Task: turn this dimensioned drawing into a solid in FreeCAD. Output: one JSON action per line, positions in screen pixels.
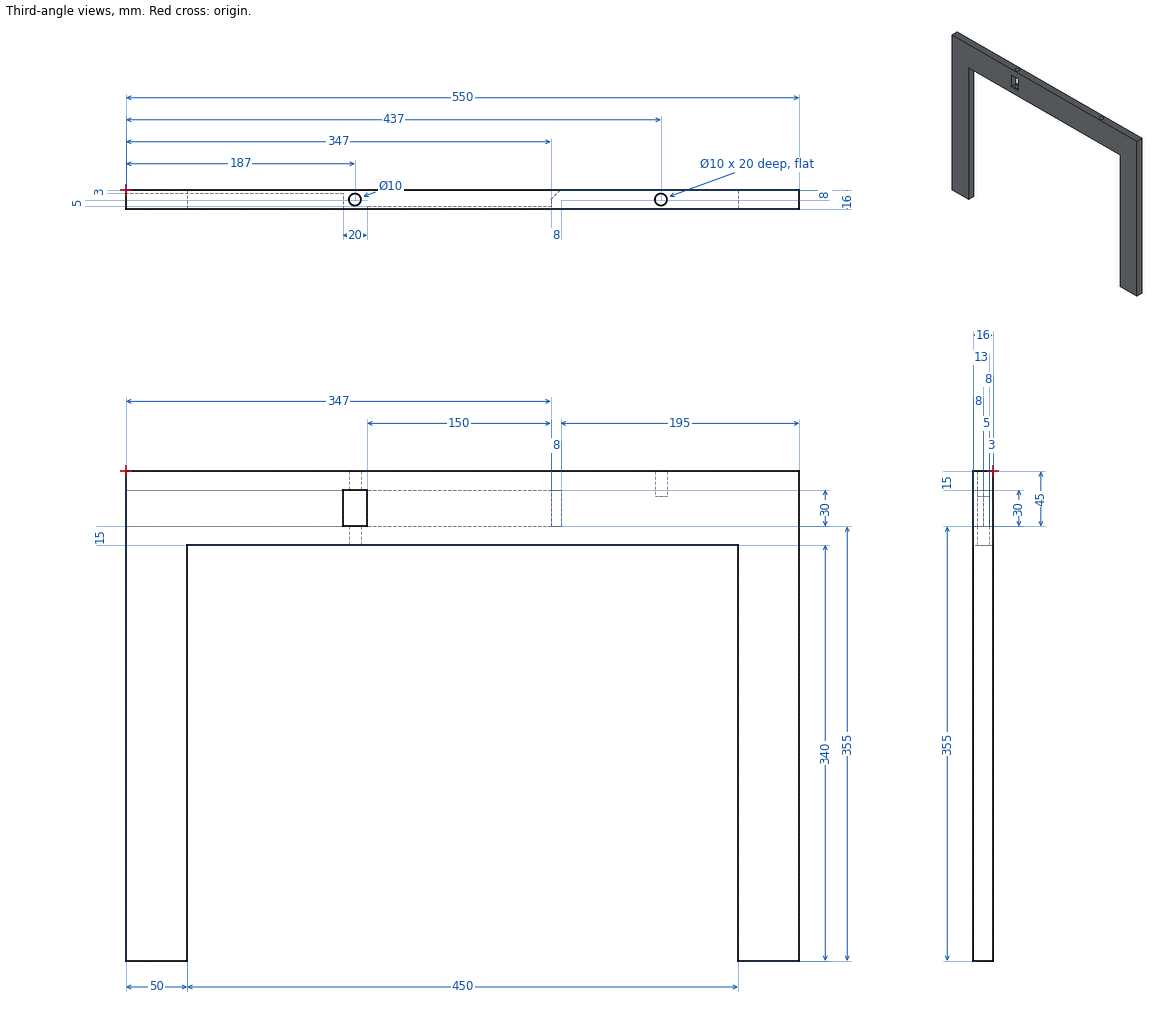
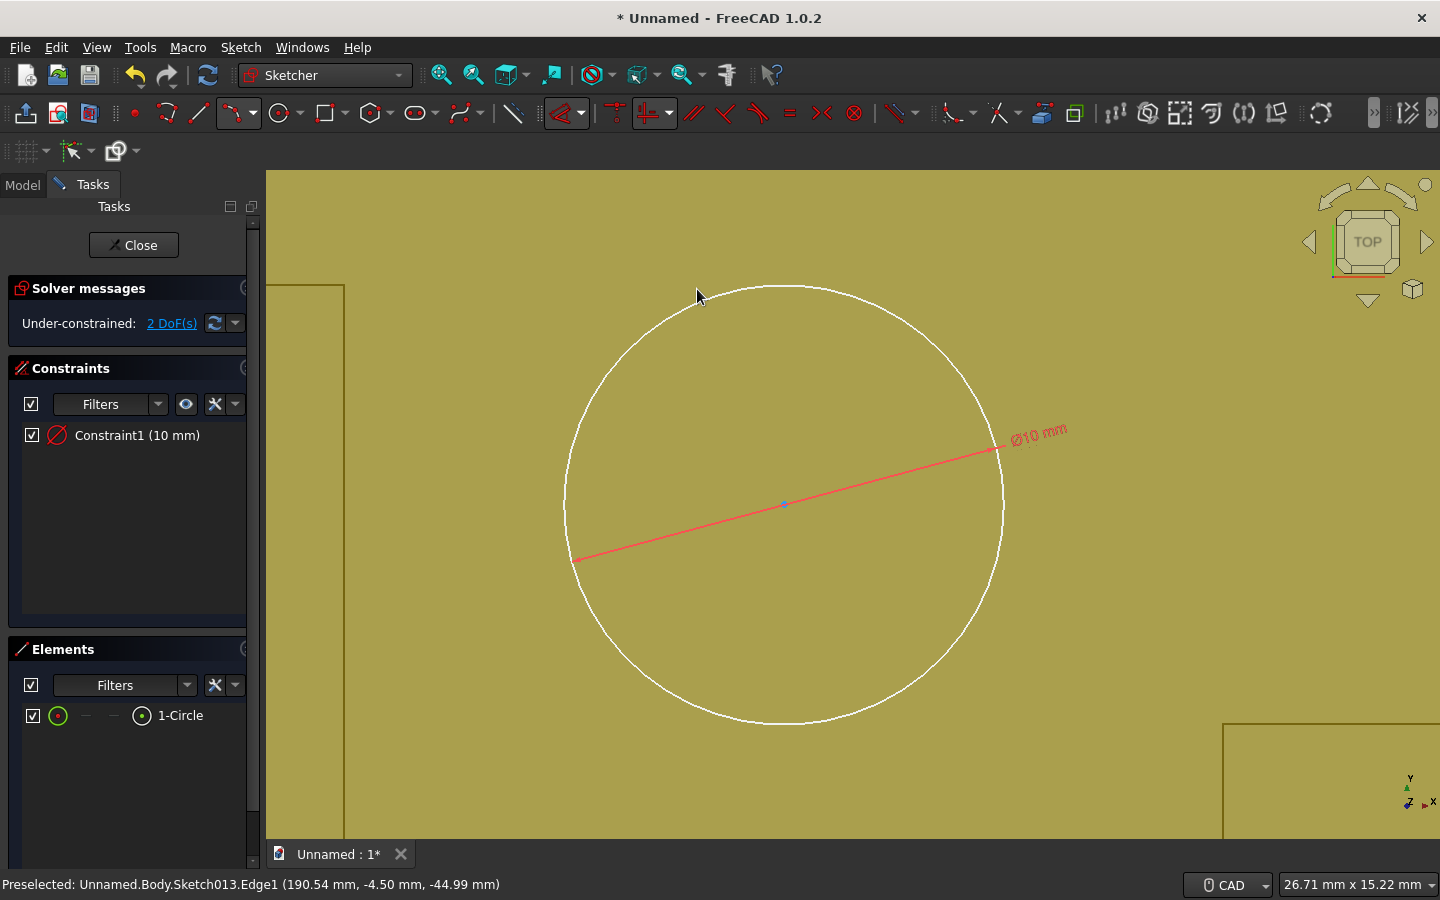
{"action": "left_click", "coordinate": [784, 505]}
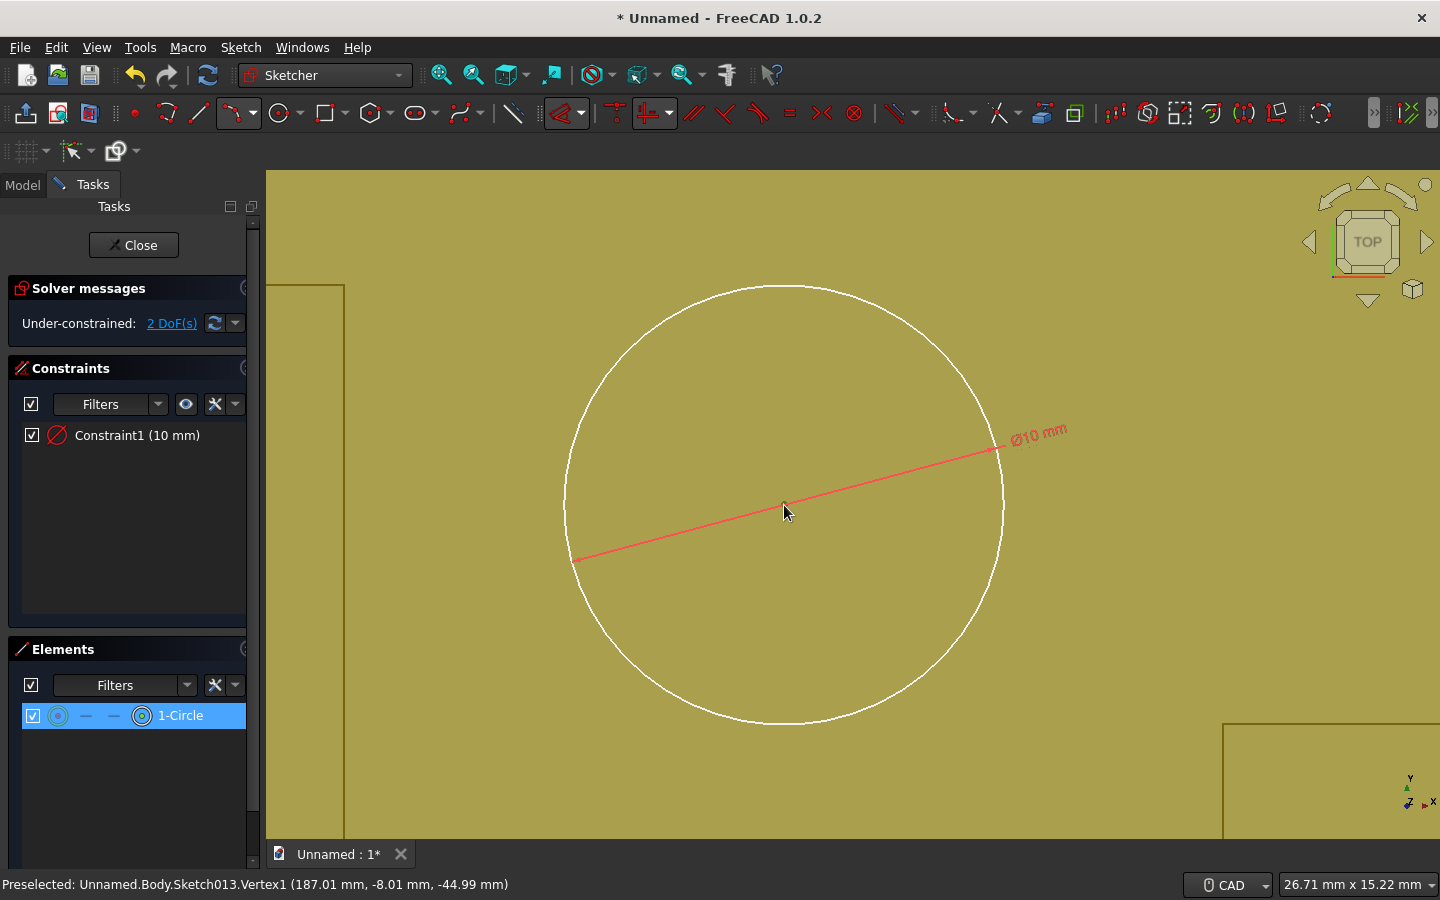
{"action": "key", "text": "i"}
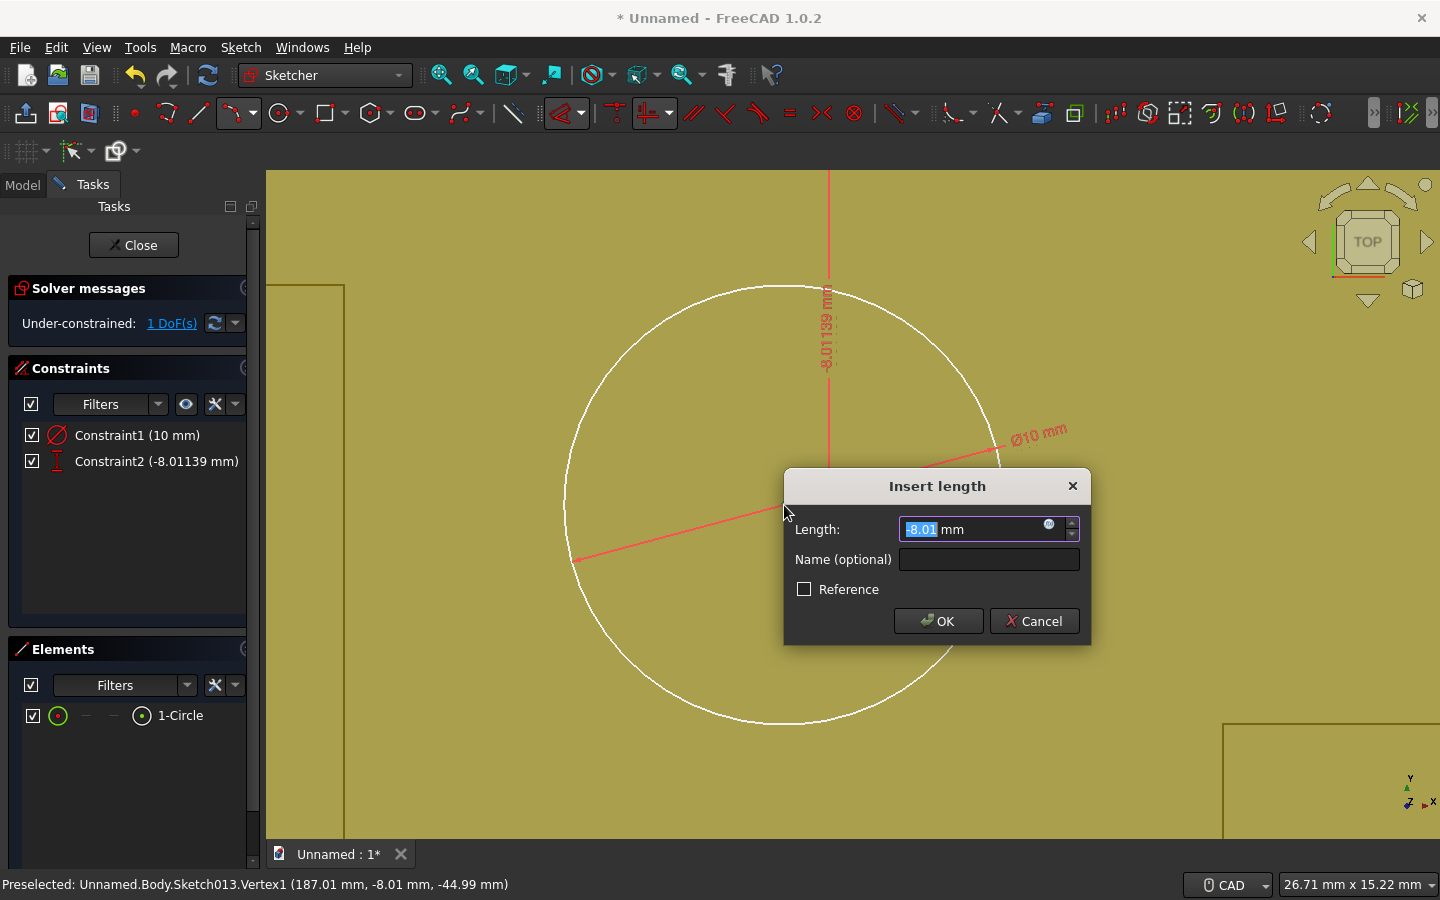
{"action": "type", "text": "-8"}
{"action": "key", "text": "Return"}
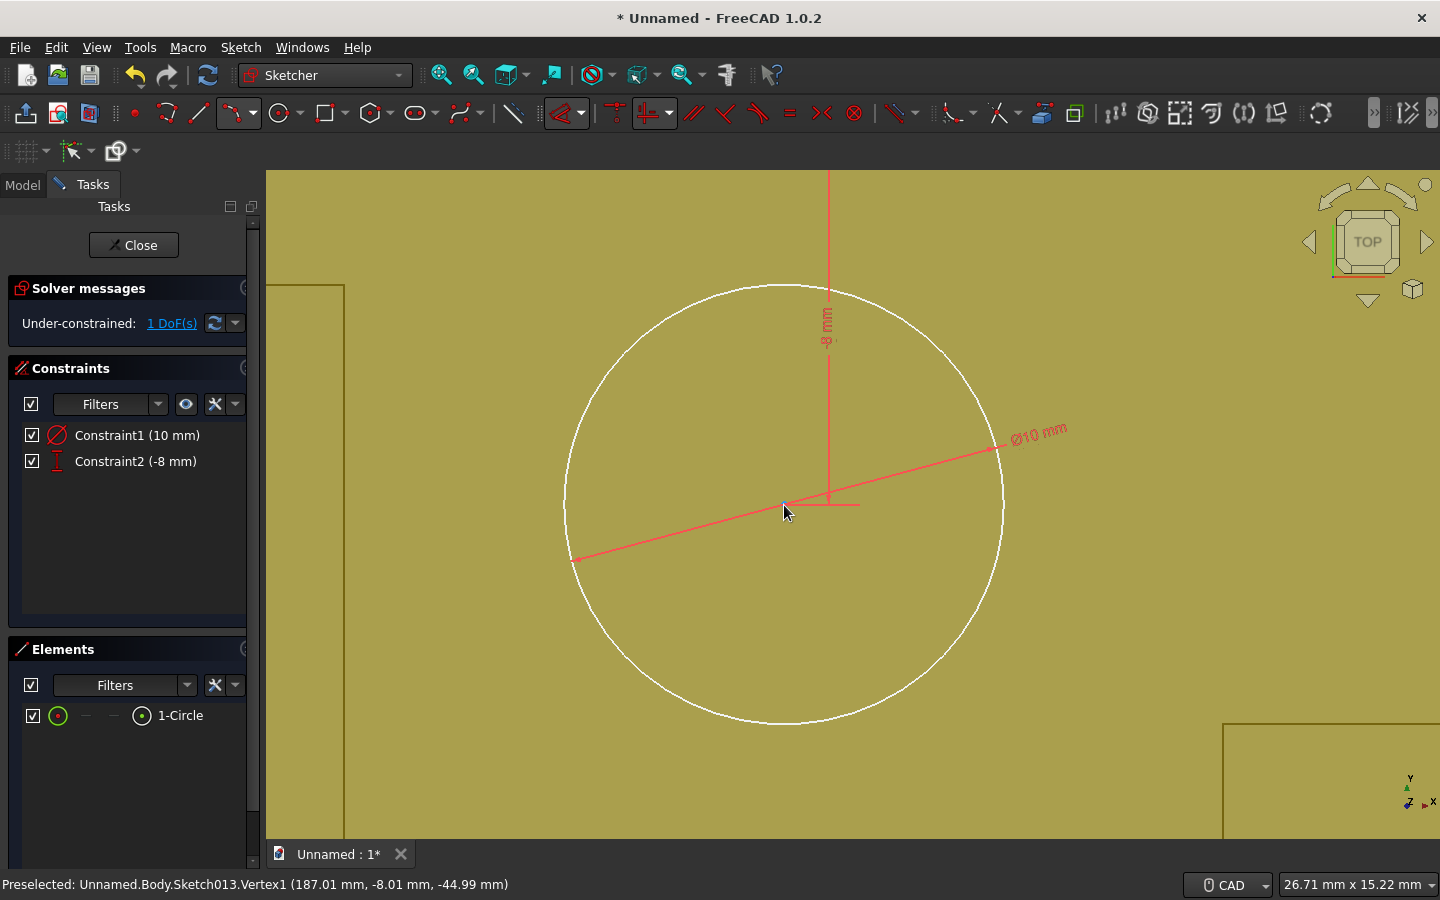
{"action": "left_click", "coordinate": [784, 504]}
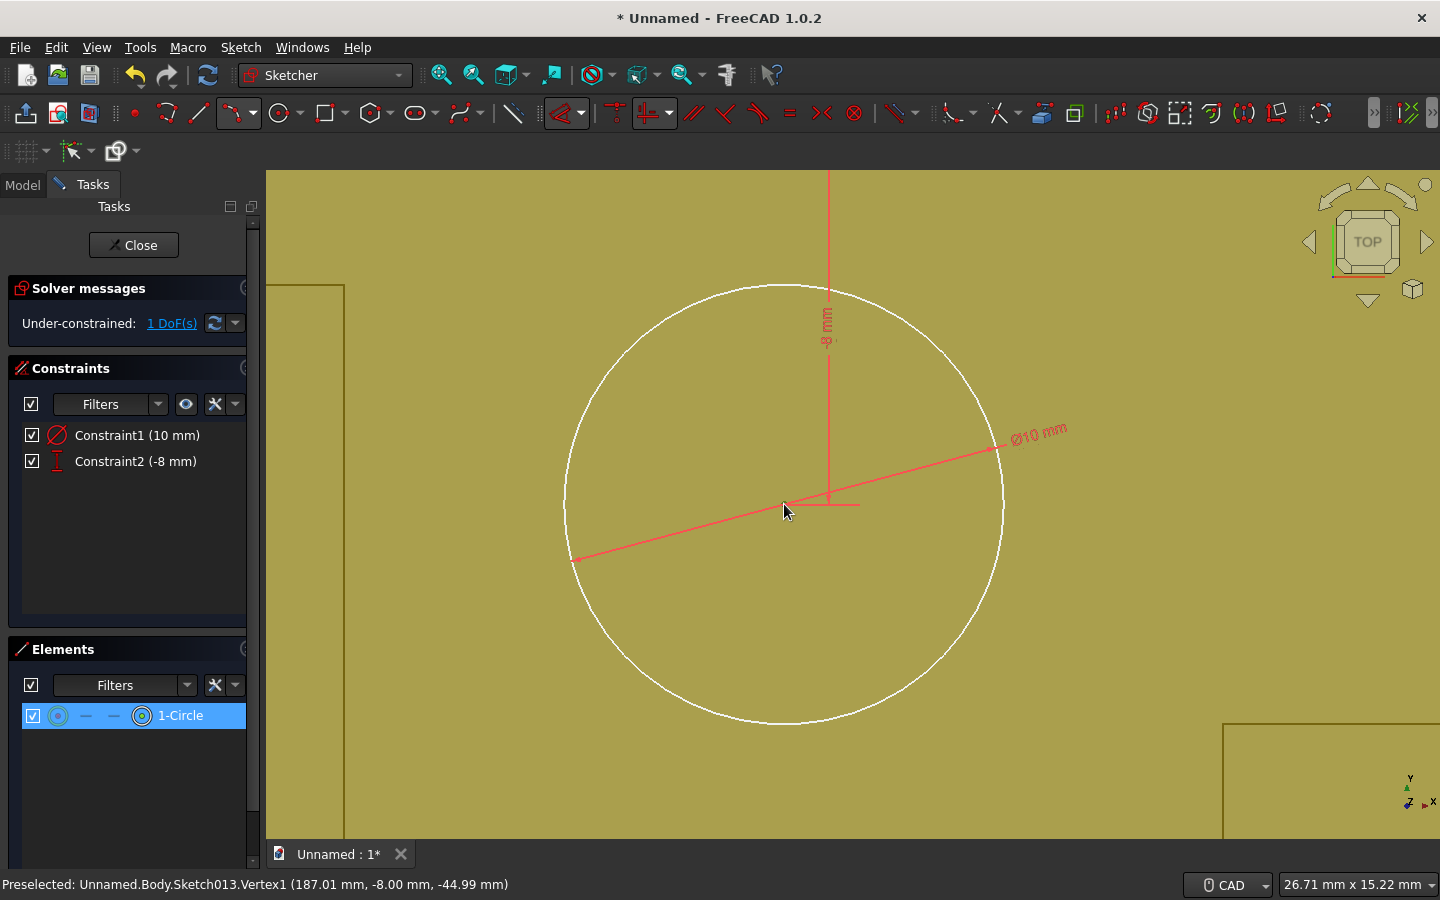
{"action": "key", "text": "l"}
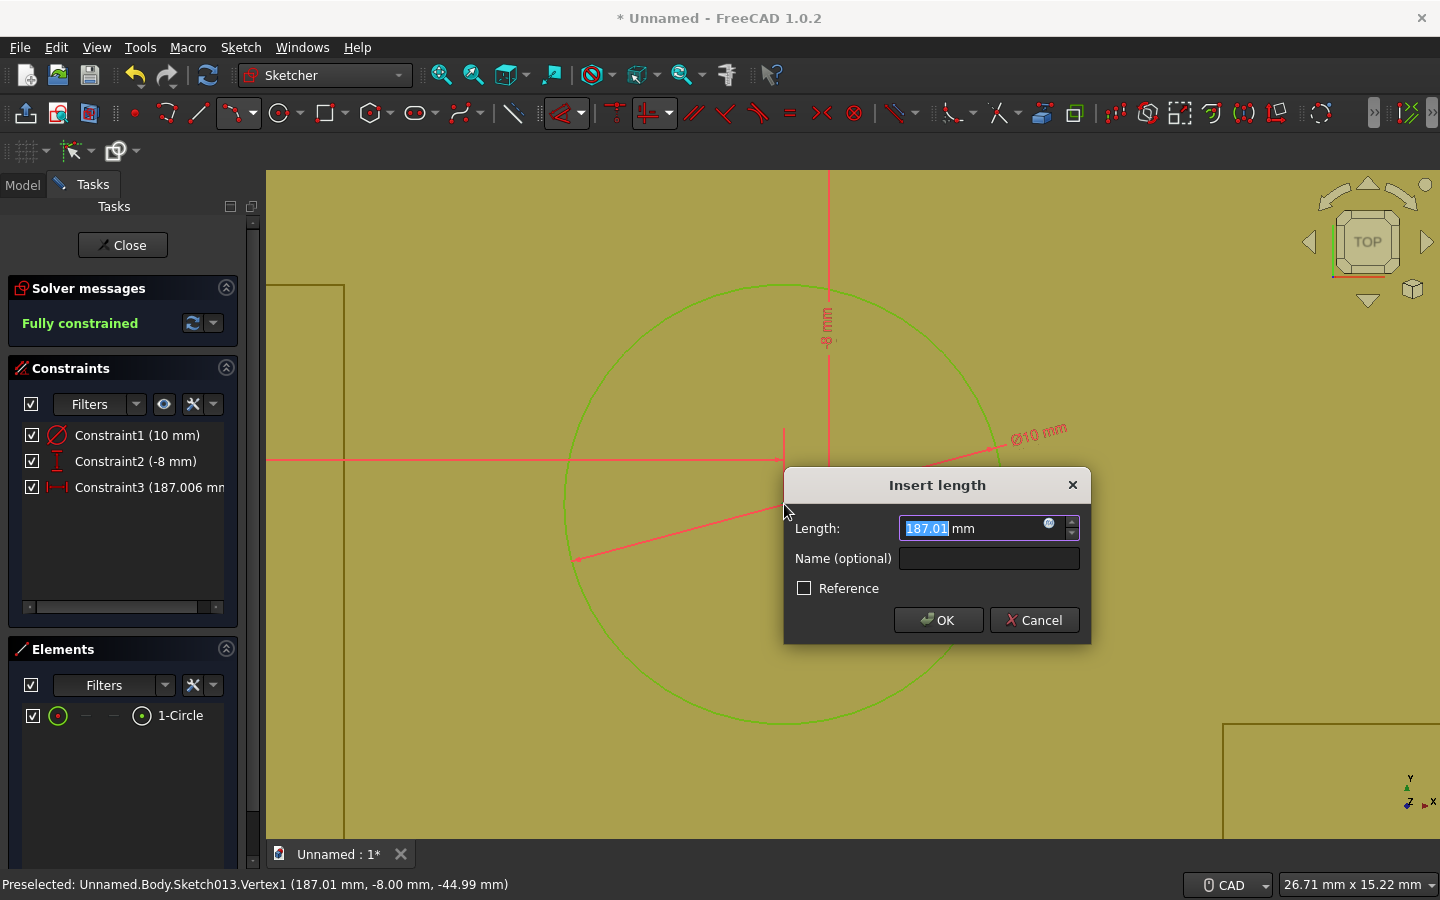
{"action": "type", "text": "187"}
{"action": "key", "text": "Return"}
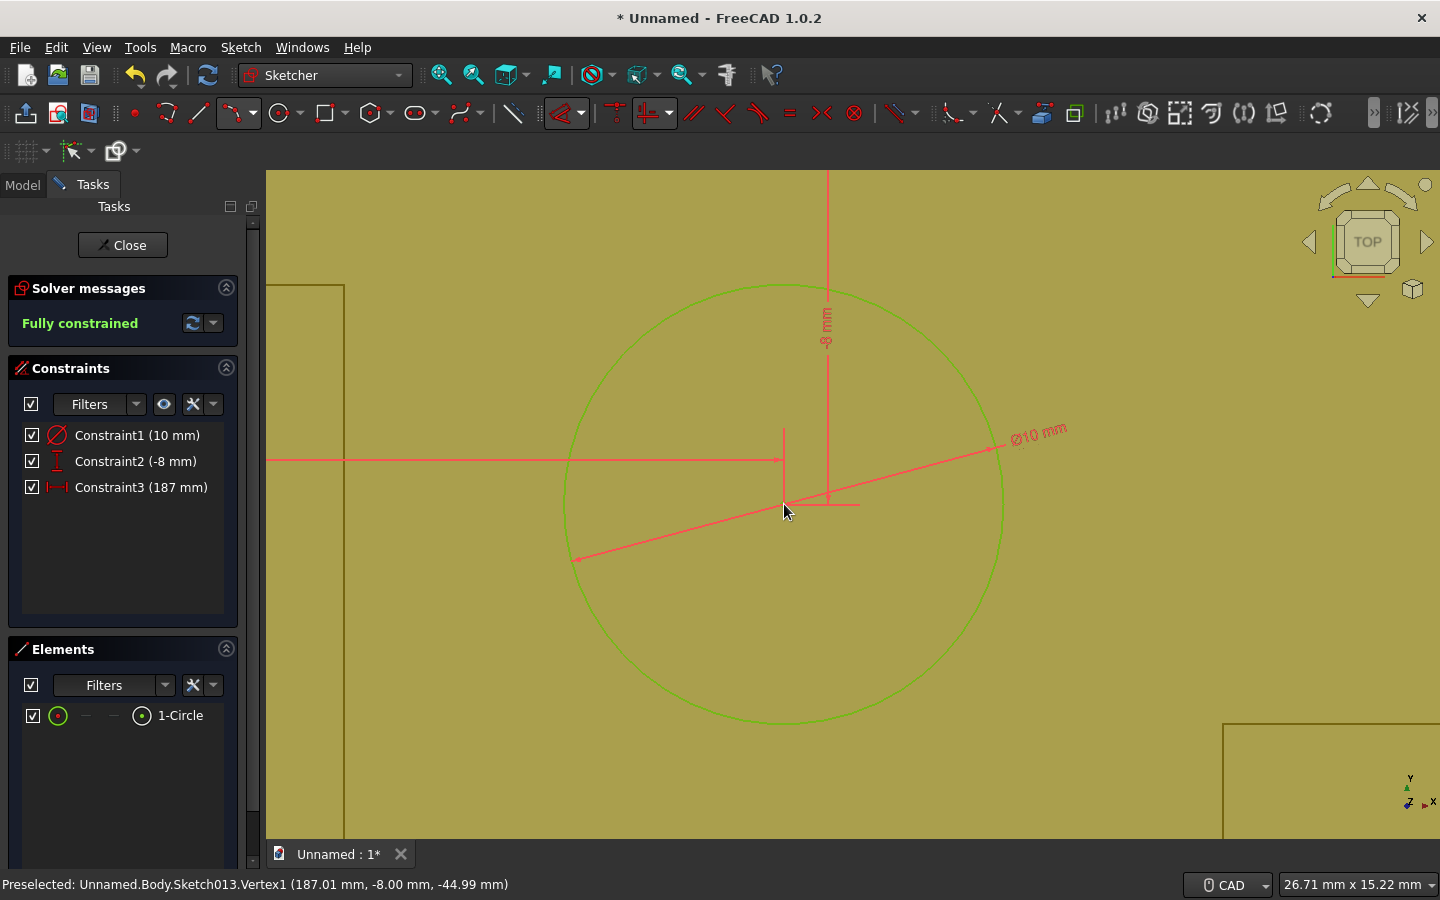
{"action": "left_click", "coordinate": [123, 245]}